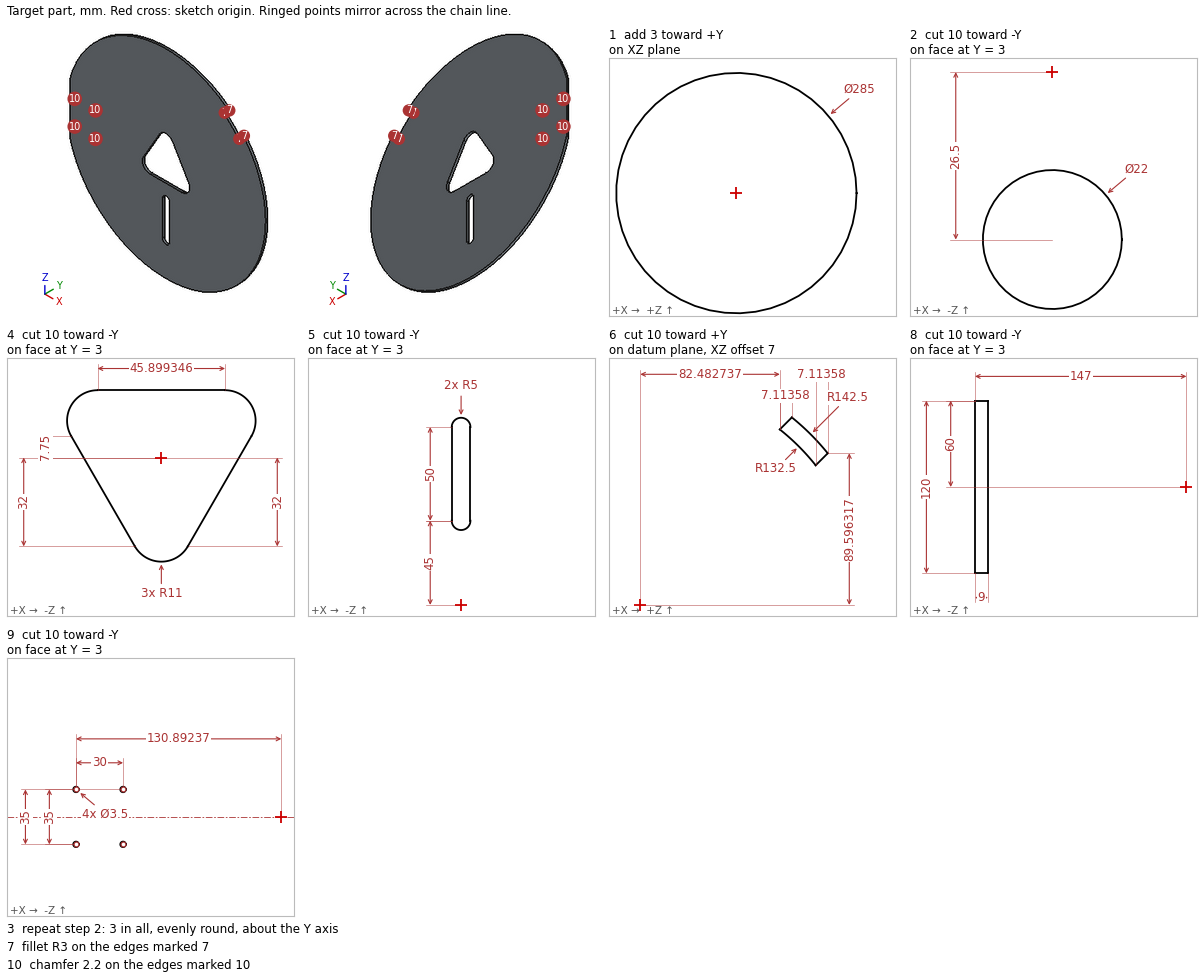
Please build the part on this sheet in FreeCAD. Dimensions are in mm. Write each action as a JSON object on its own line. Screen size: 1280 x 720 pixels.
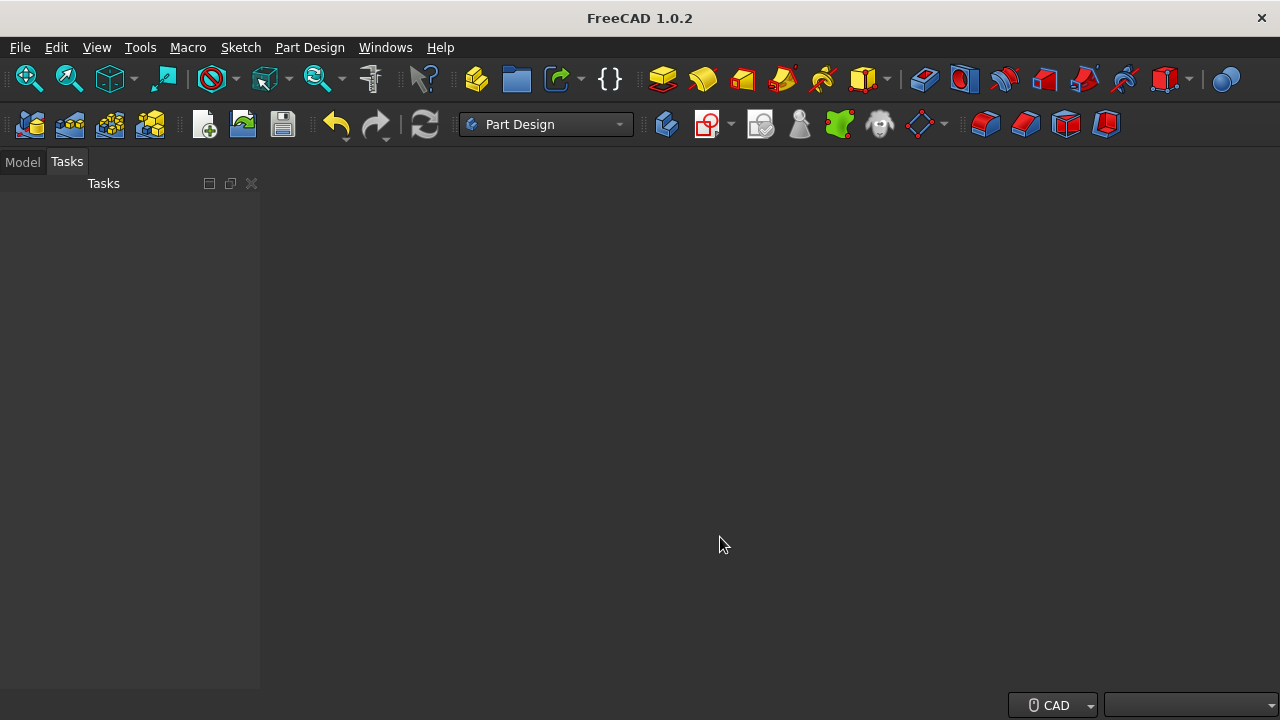
{"action": "key", "text": "ctrl+n"}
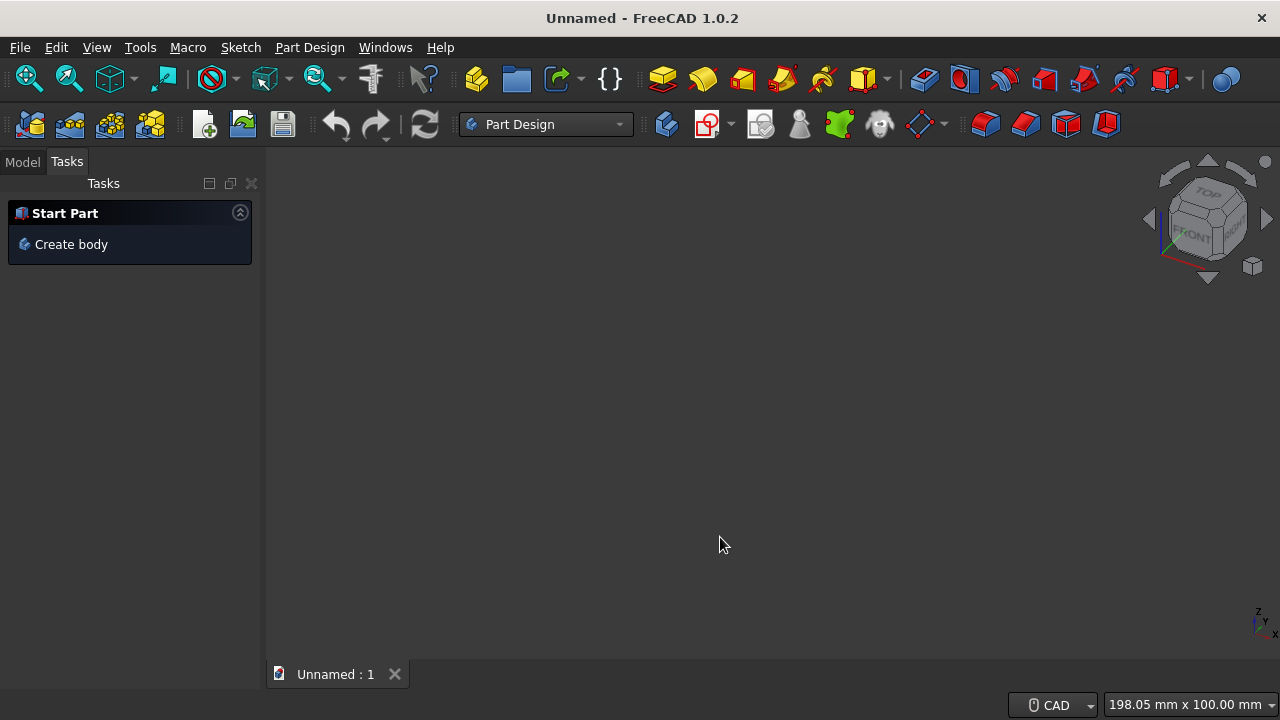
{"action": "left_click", "coordinate": [708, 124]}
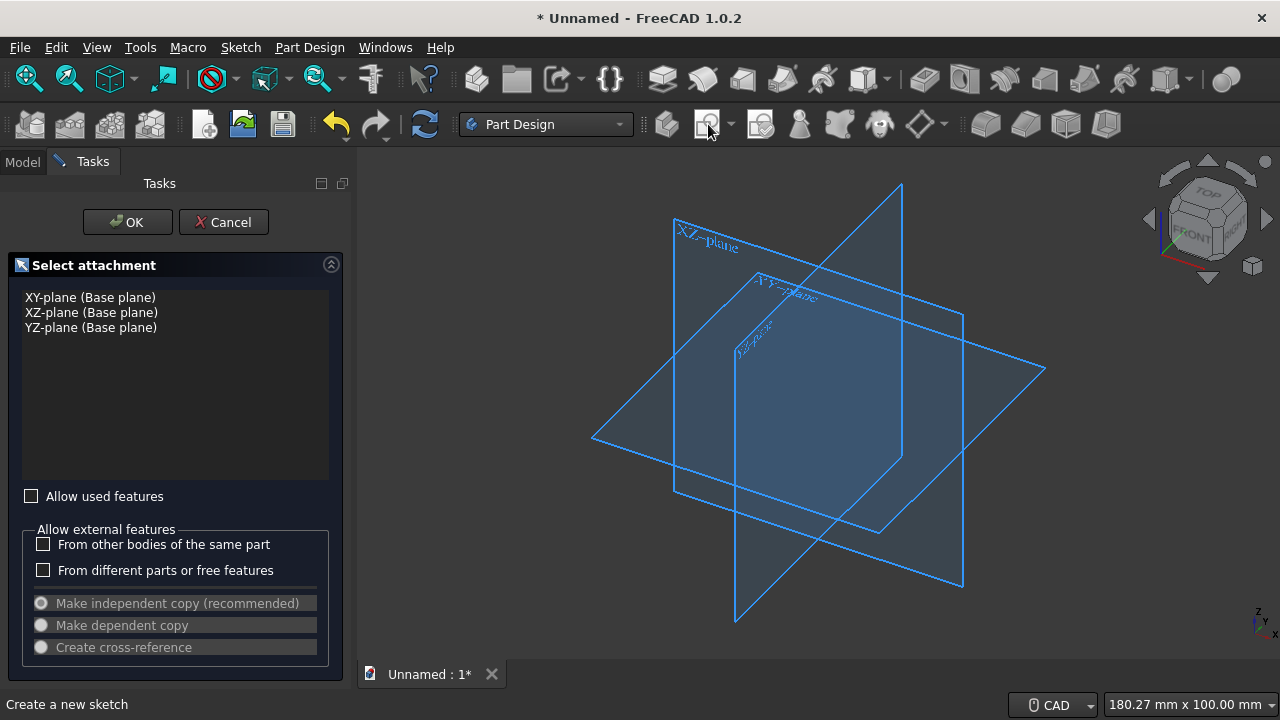
{"action": "left_click", "coordinate": [82, 312]}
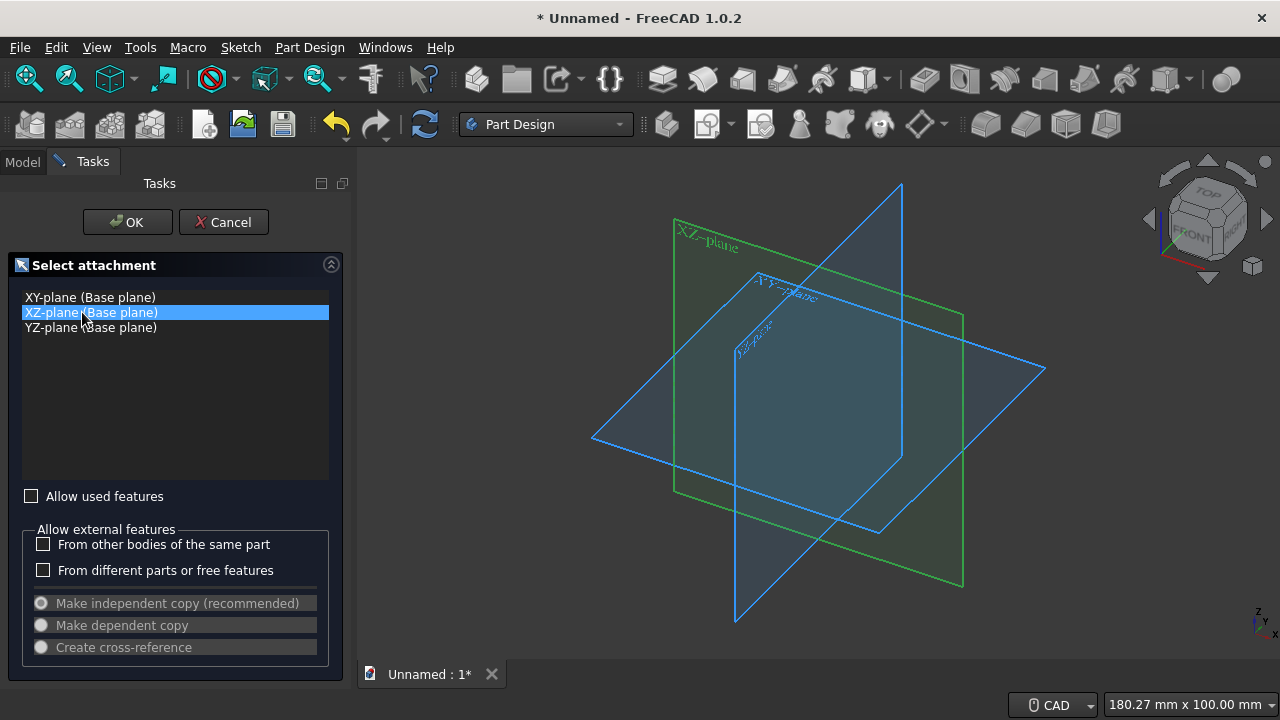
{"action": "left_click", "coordinate": [128, 222]}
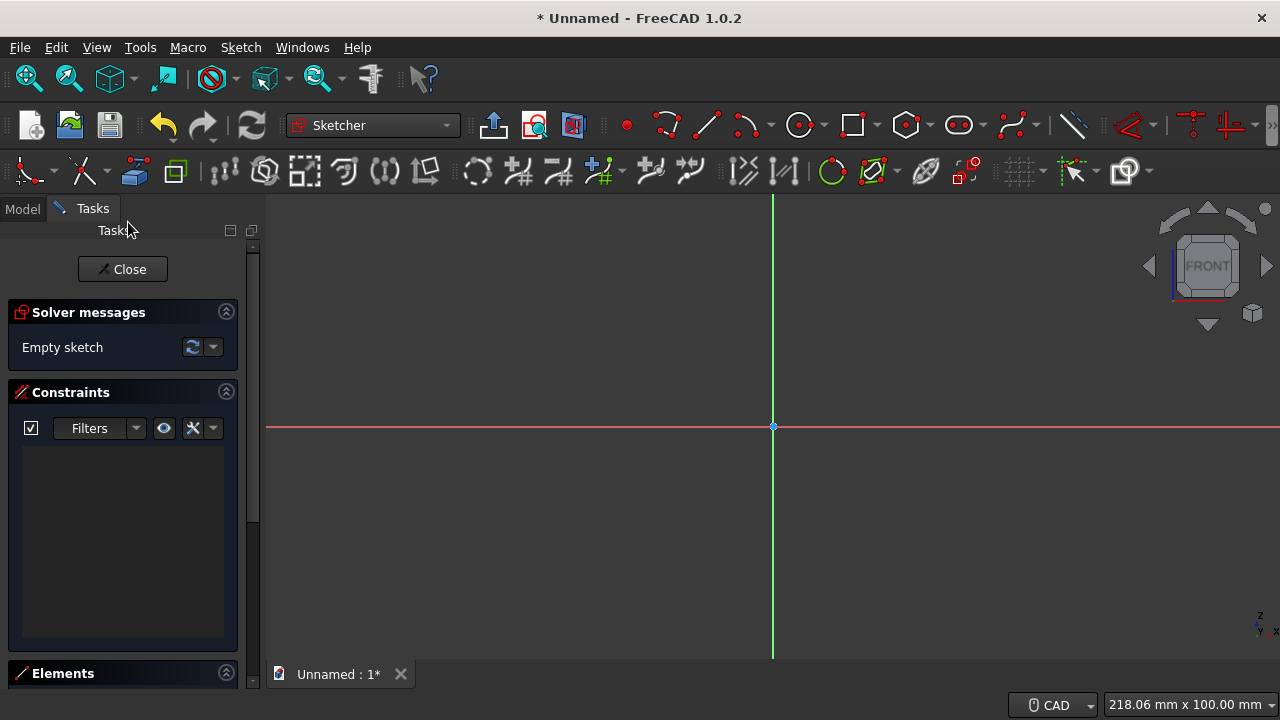
{"action": "scroll", "coordinate": [687, 426], "scroll_direction": "down", "scroll_amount": 8}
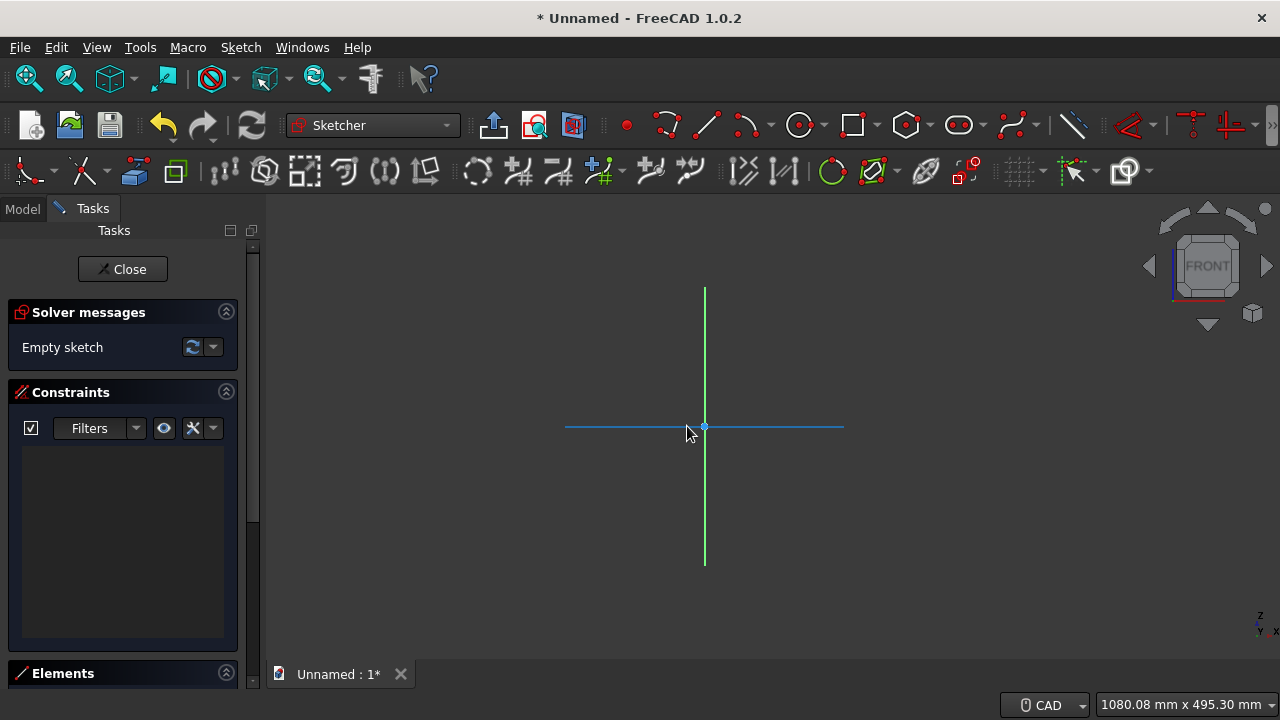
{"action": "left_click", "coordinate": [800, 126]}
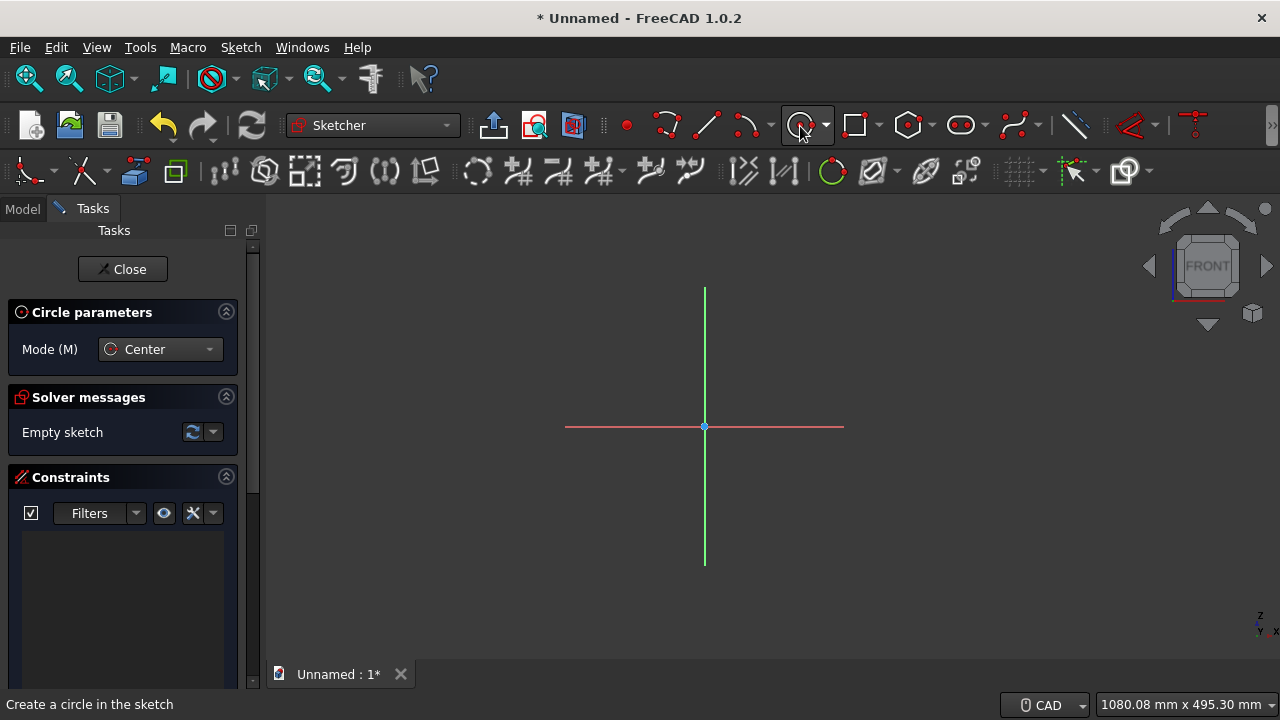
{"action": "left_click", "coordinate": [705, 426]}
{"action": "left_click", "coordinate": [799, 332]}
{"action": "key", "text": "Escape"}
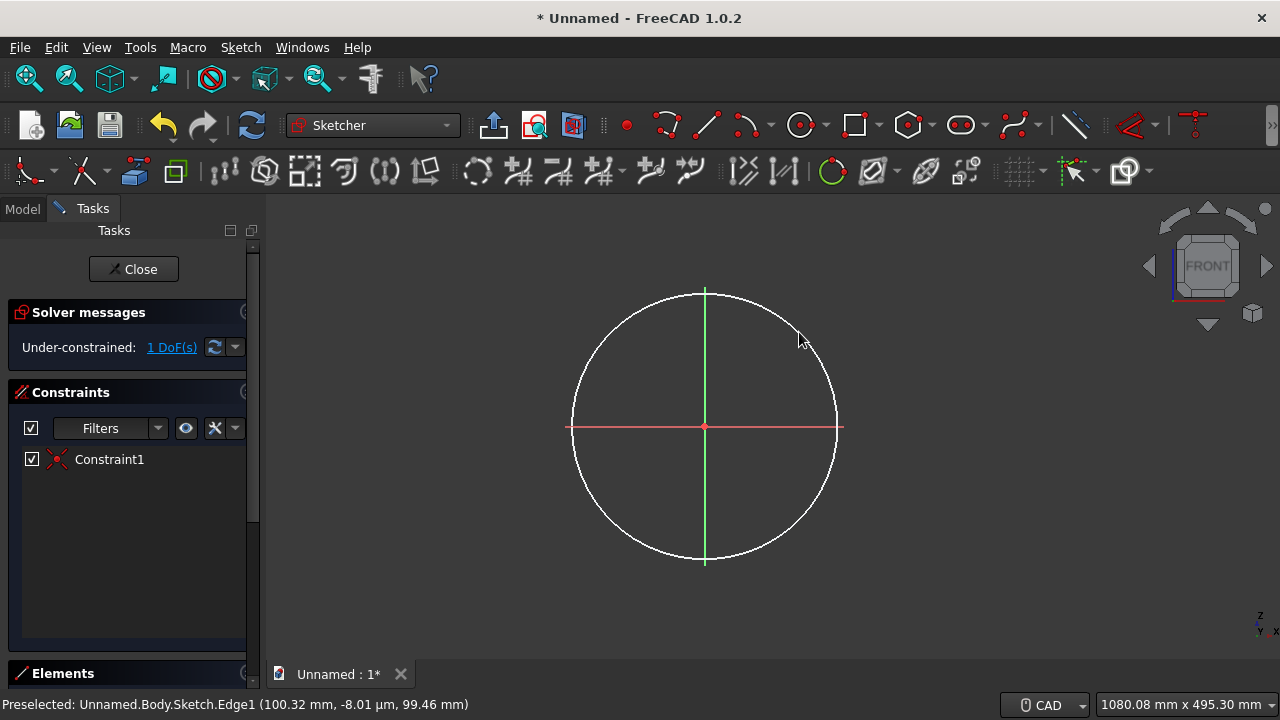
{"action": "left_click", "coordinate": [798, 332]}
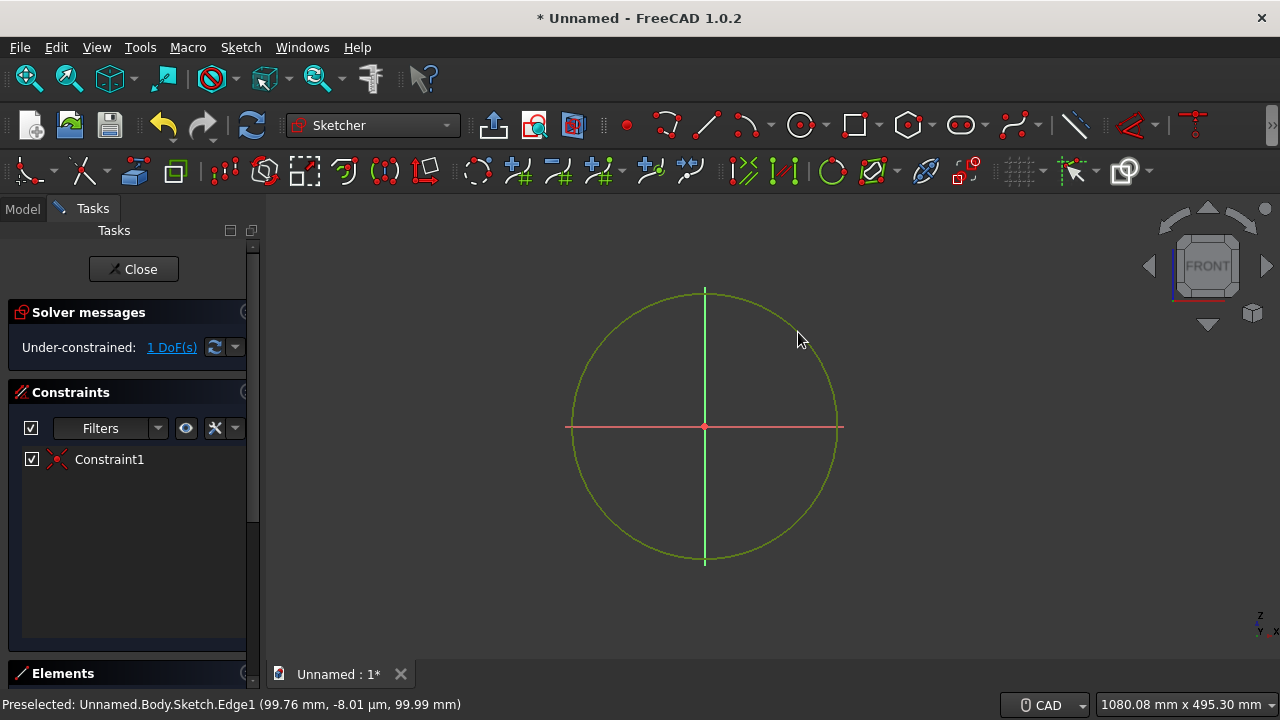
{"action": "key", "text": "k o"}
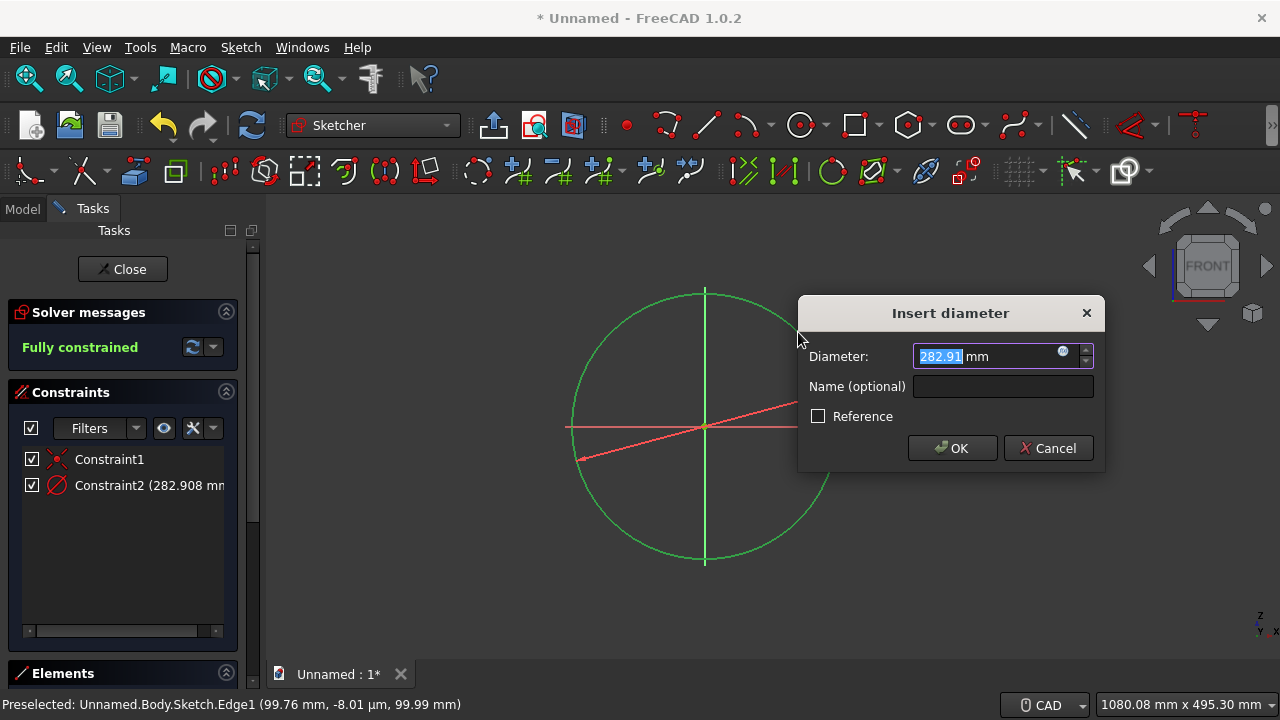
{"action": "type", "text": "285"}
{"action": "key", "text": "Return"}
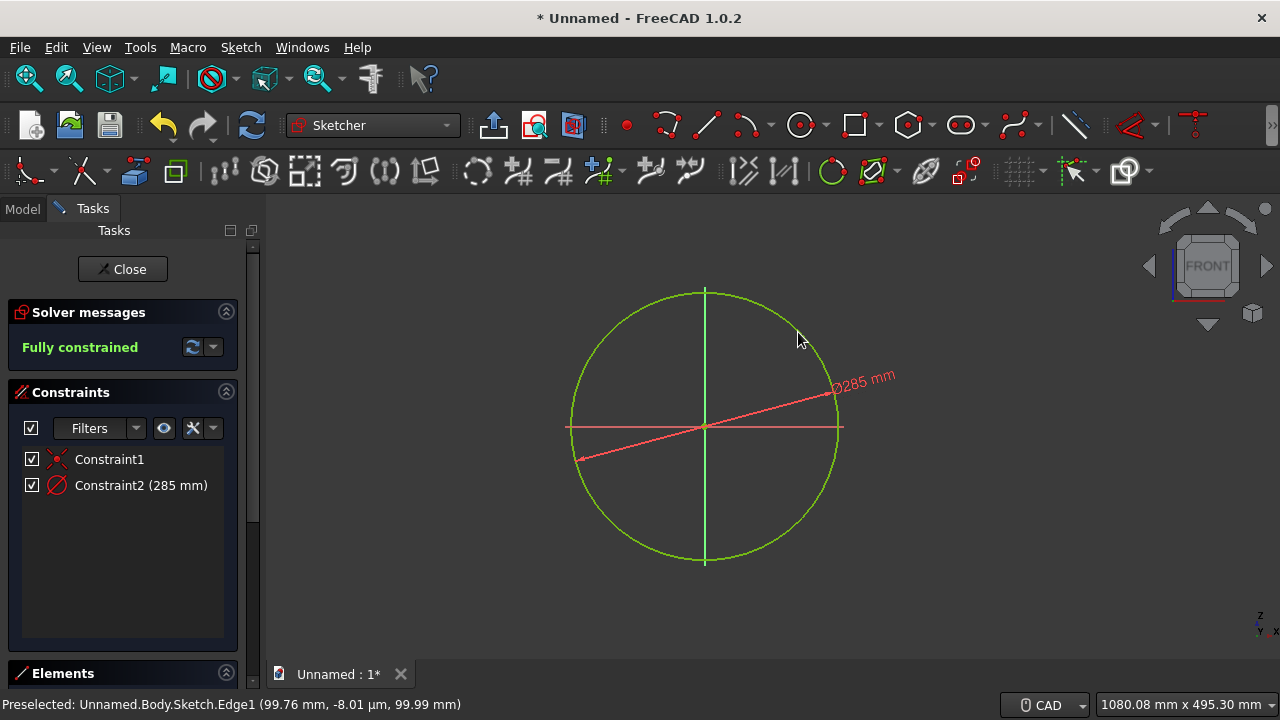
{"action": "left_click", "coordinate": [123, 269]}